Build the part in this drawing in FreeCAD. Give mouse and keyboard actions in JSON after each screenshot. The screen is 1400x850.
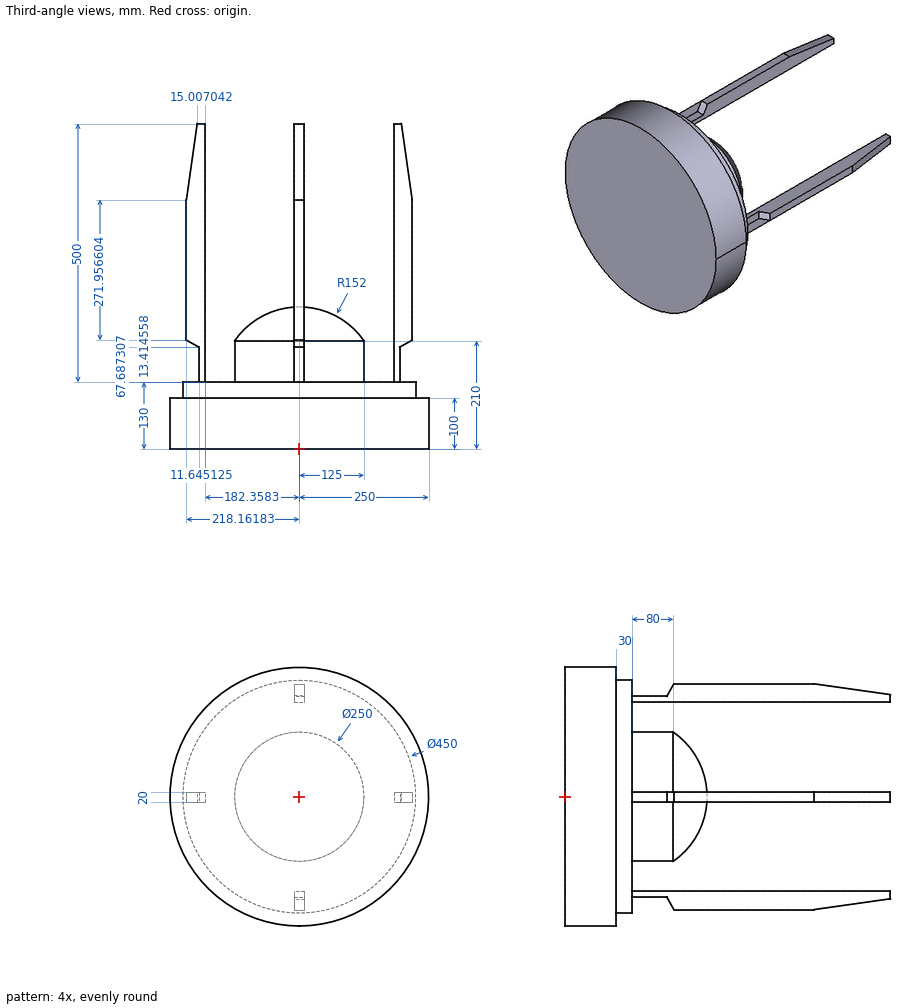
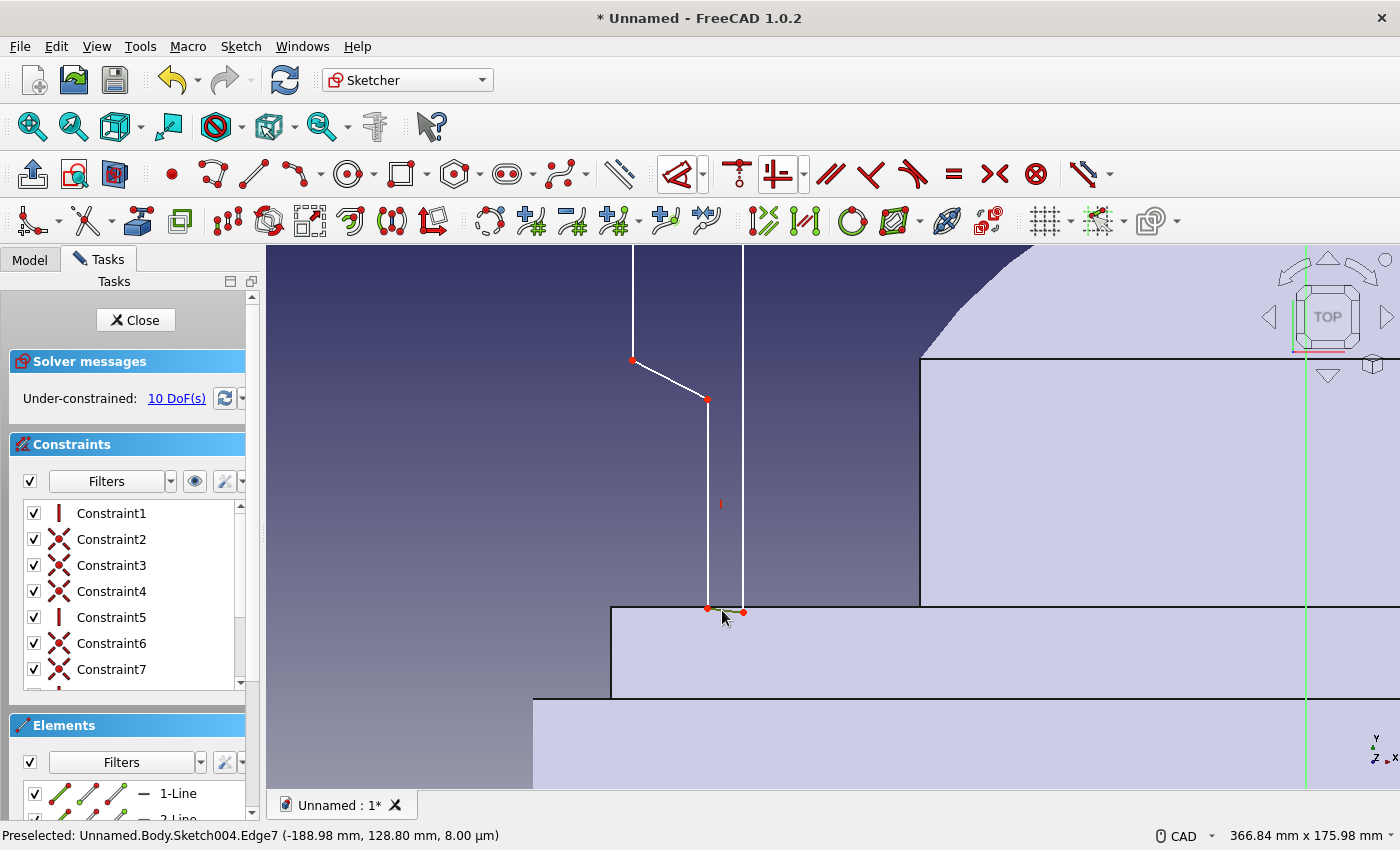
{"action": "key", "text": "h"}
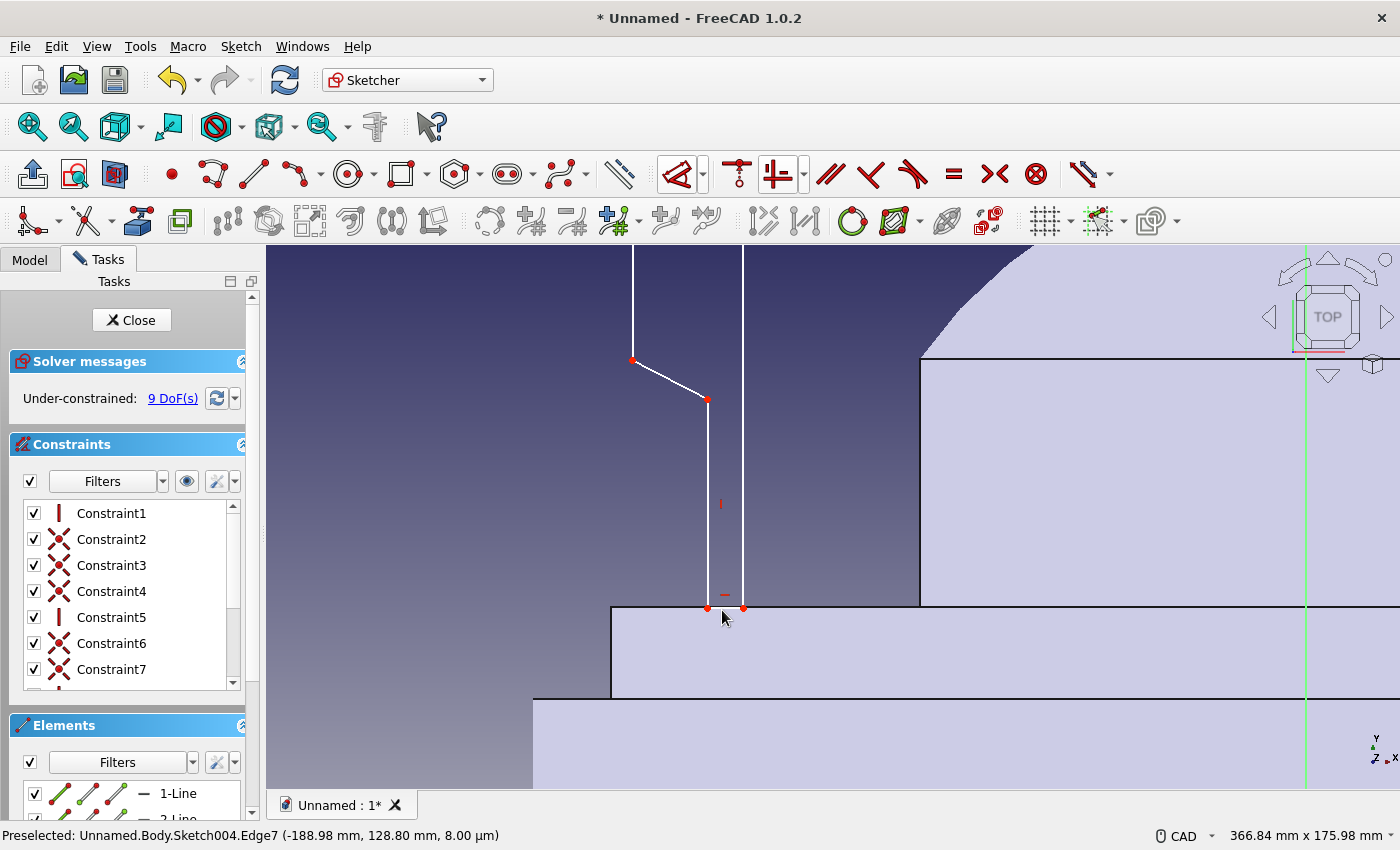
{"action": "scroll", "coordinate": [724, 613], "scroll_direction": "down", "scroll_amount": 9}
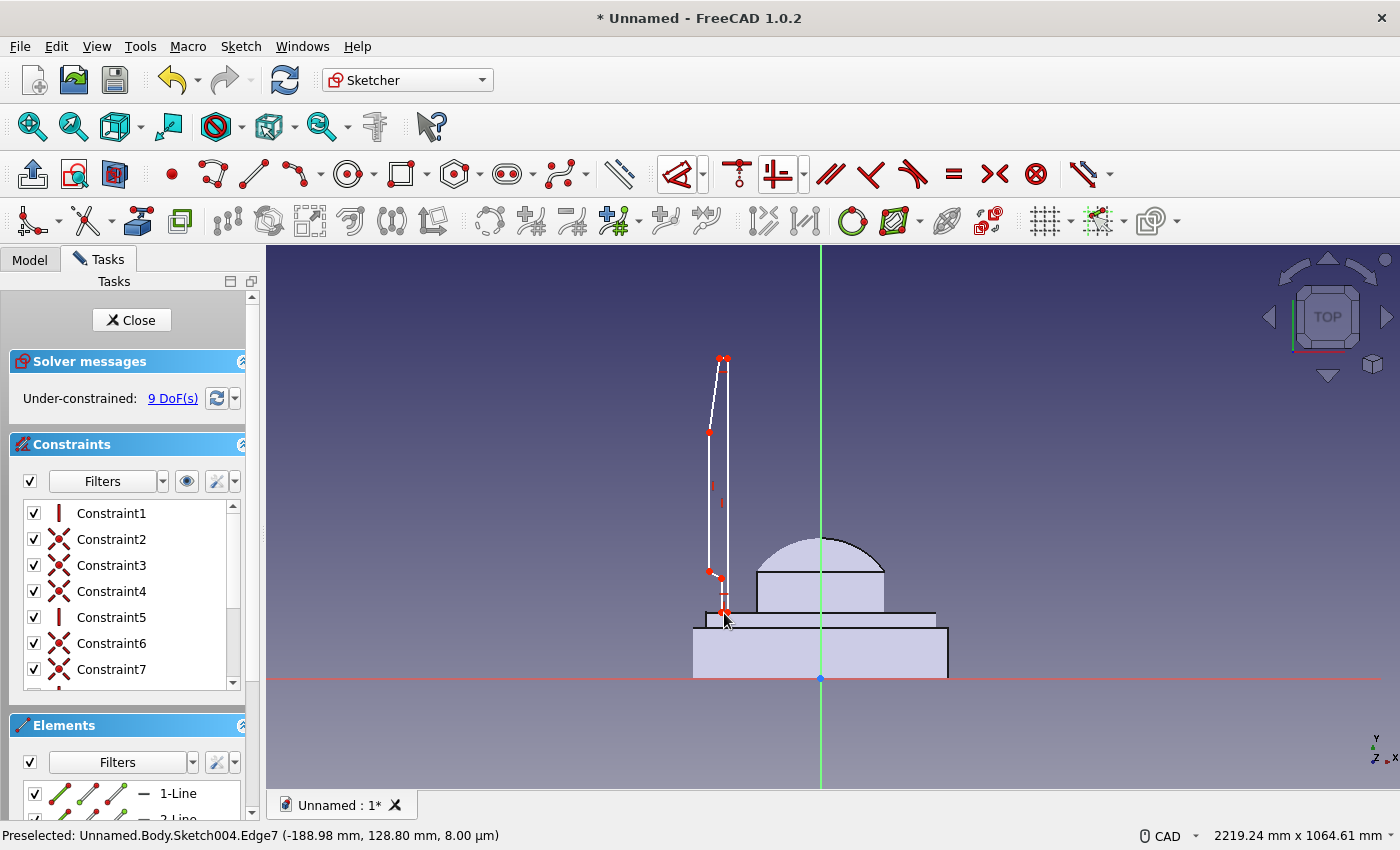
{"action": "left_click", "coordinate": [728, 562]}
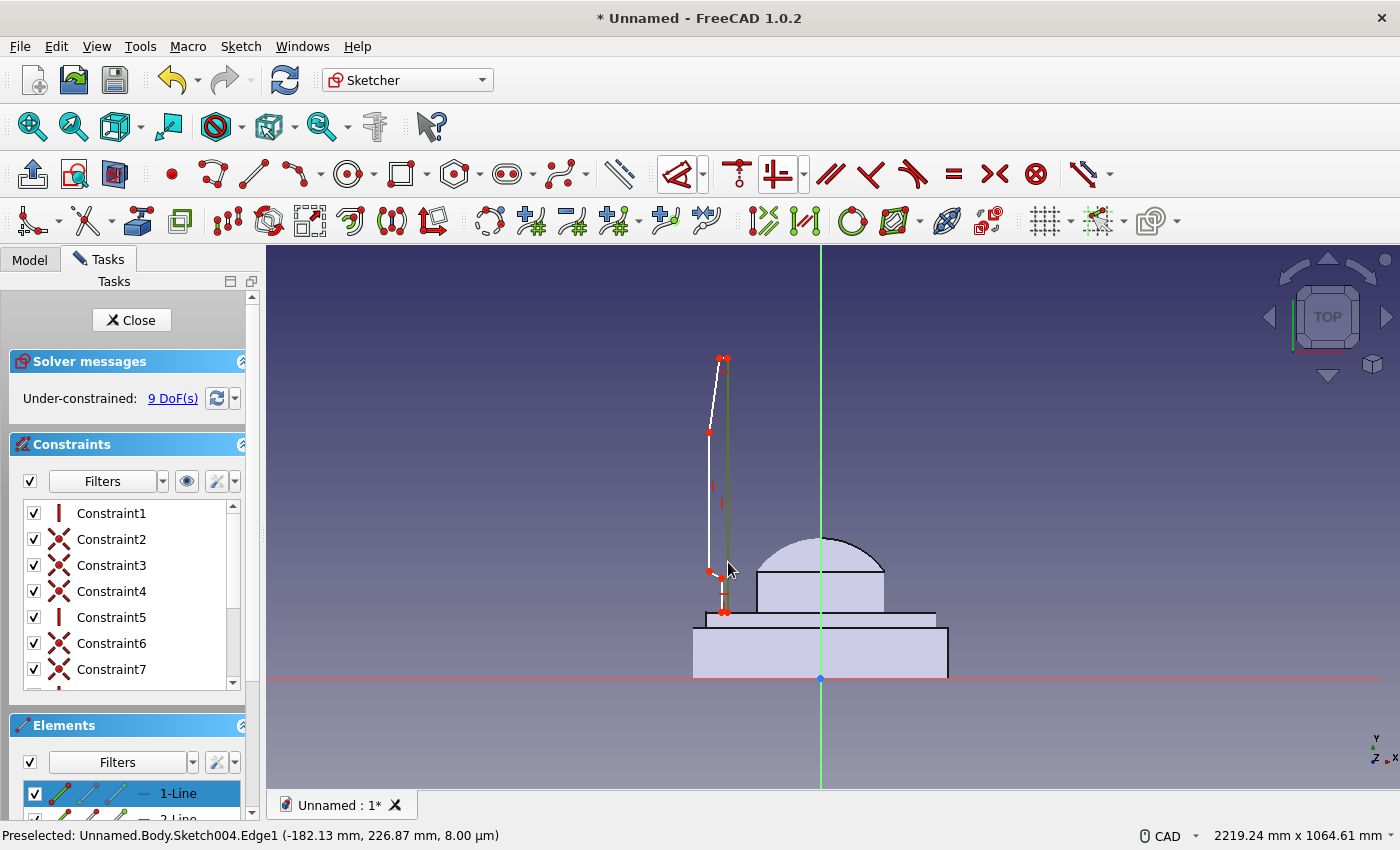
{"action": "left_click", "coordinate": [702, 174]}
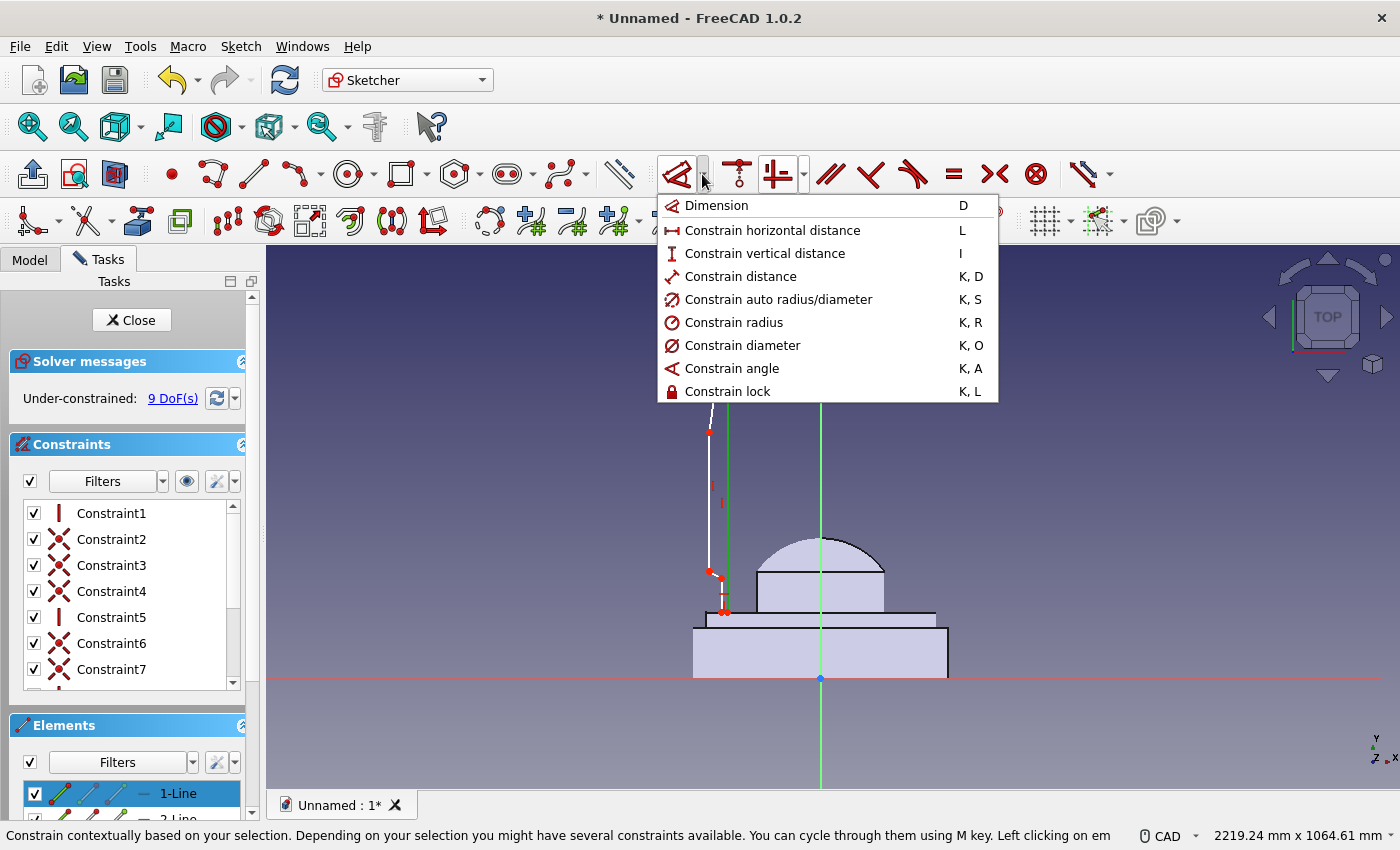
{"action": "left_click", "coordinate": [828, 254]}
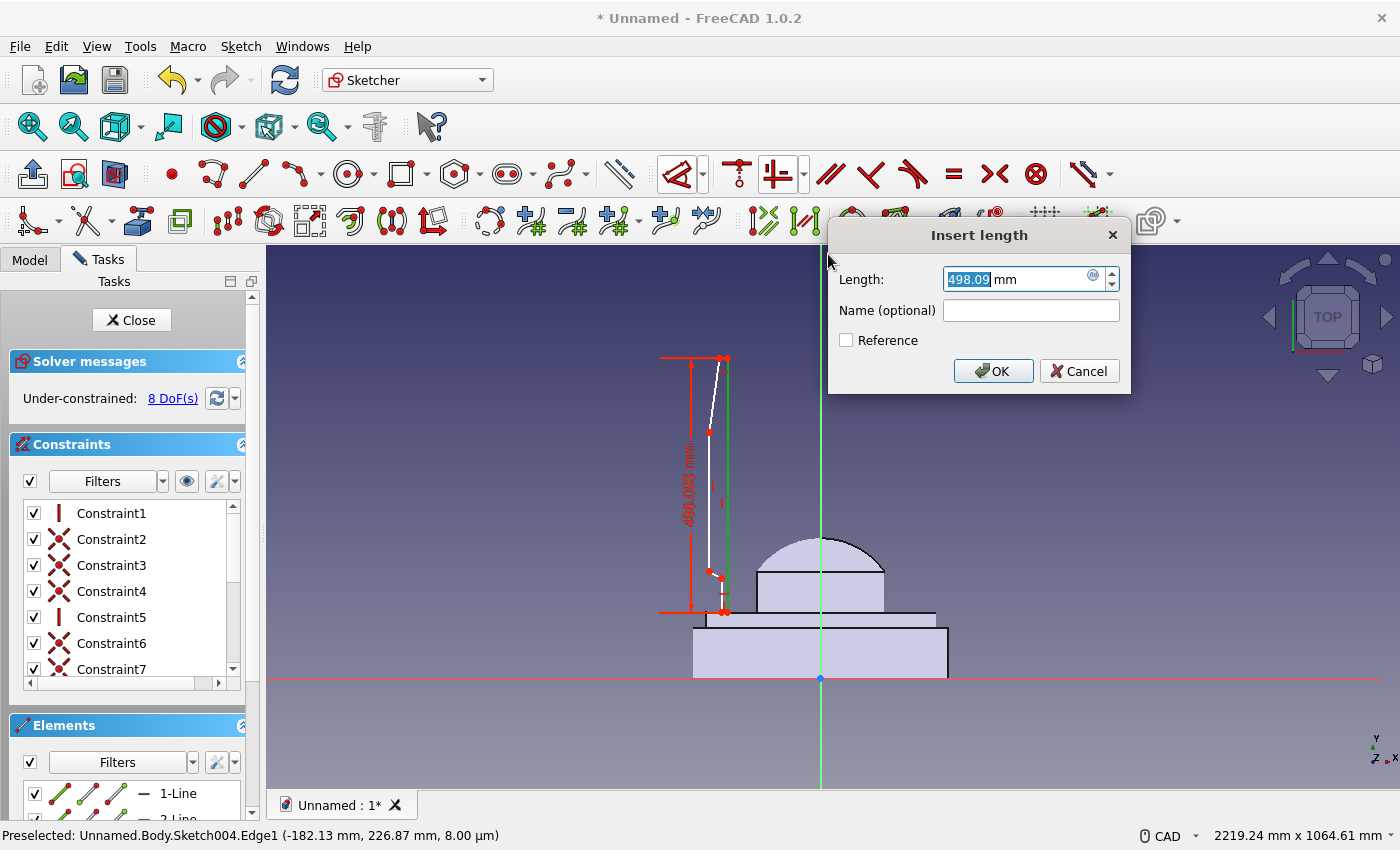
{"action": "type", "text": "500"}
{"action": "key", "text": "Return"}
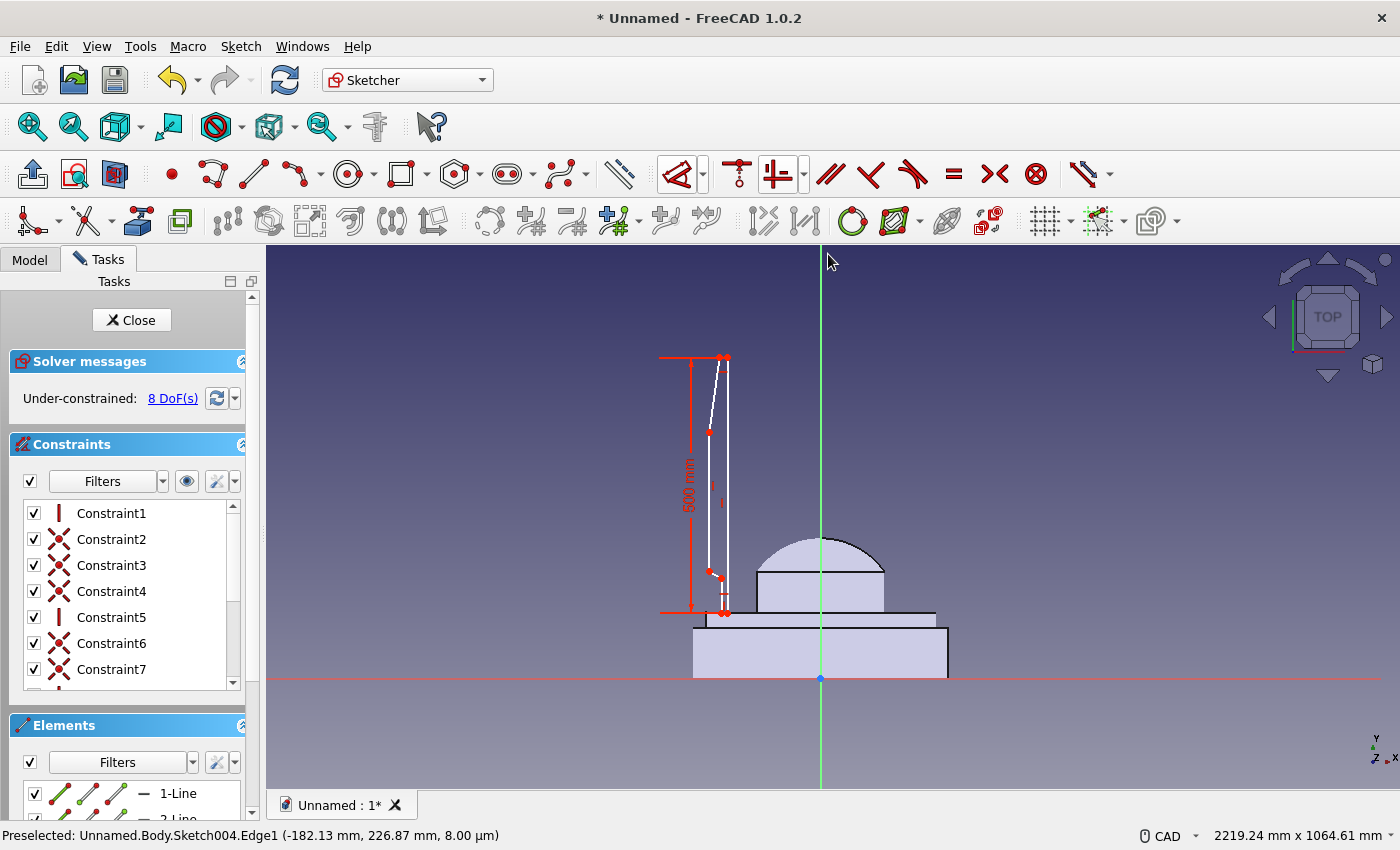
{"action": "scroll", "coordinate": [728, 613], "scroll_direction": "up", "scroll_amount": 4}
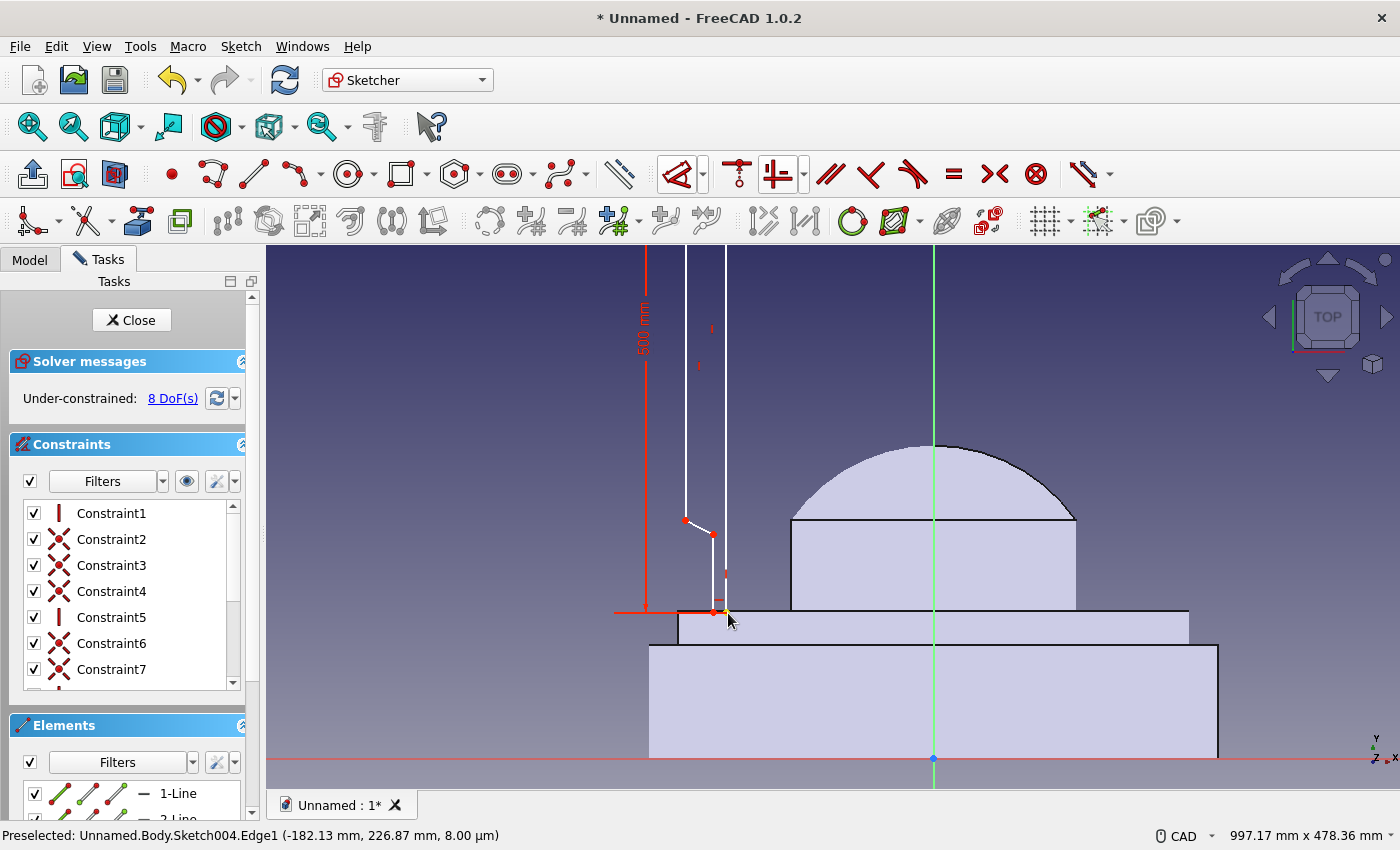
{"action": "left_click", "coordinate": [726, 613]}